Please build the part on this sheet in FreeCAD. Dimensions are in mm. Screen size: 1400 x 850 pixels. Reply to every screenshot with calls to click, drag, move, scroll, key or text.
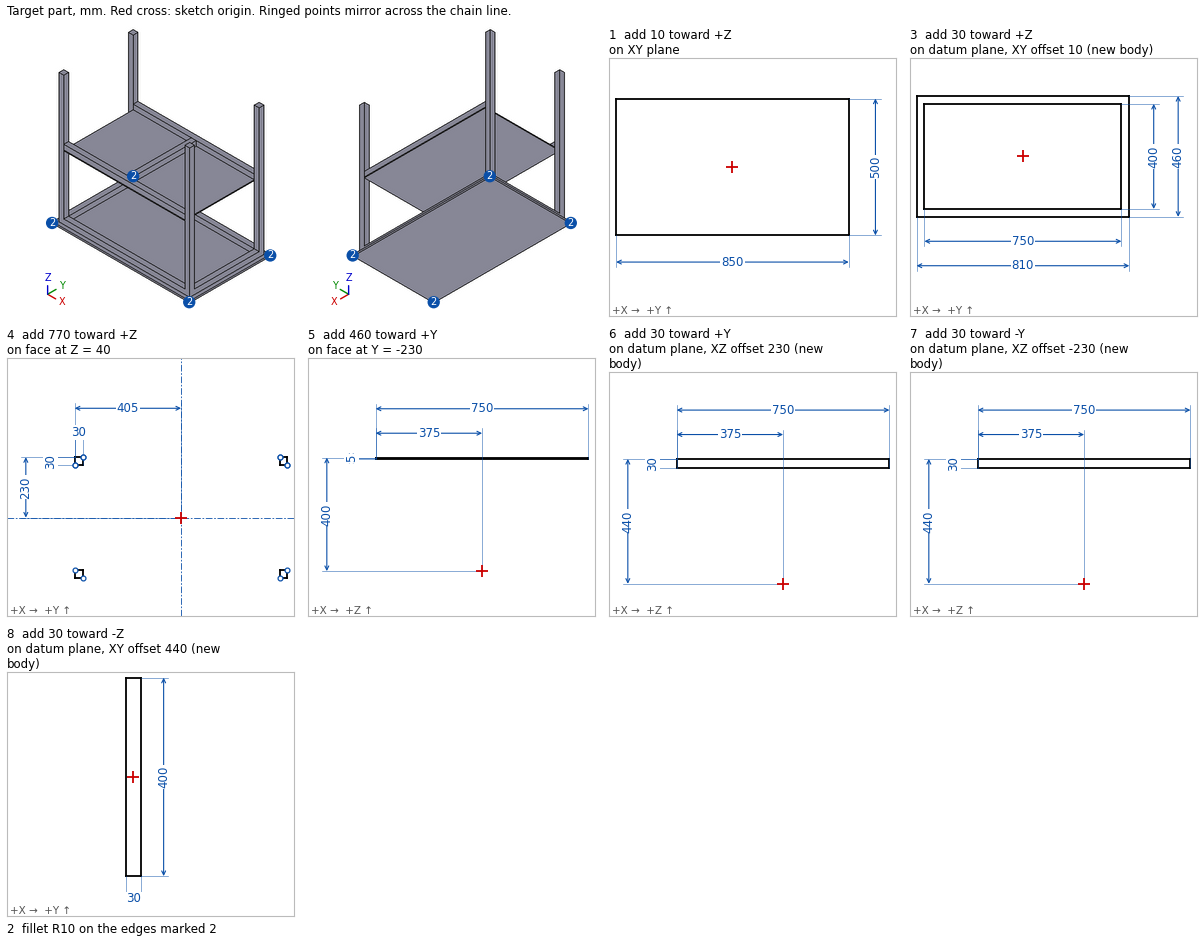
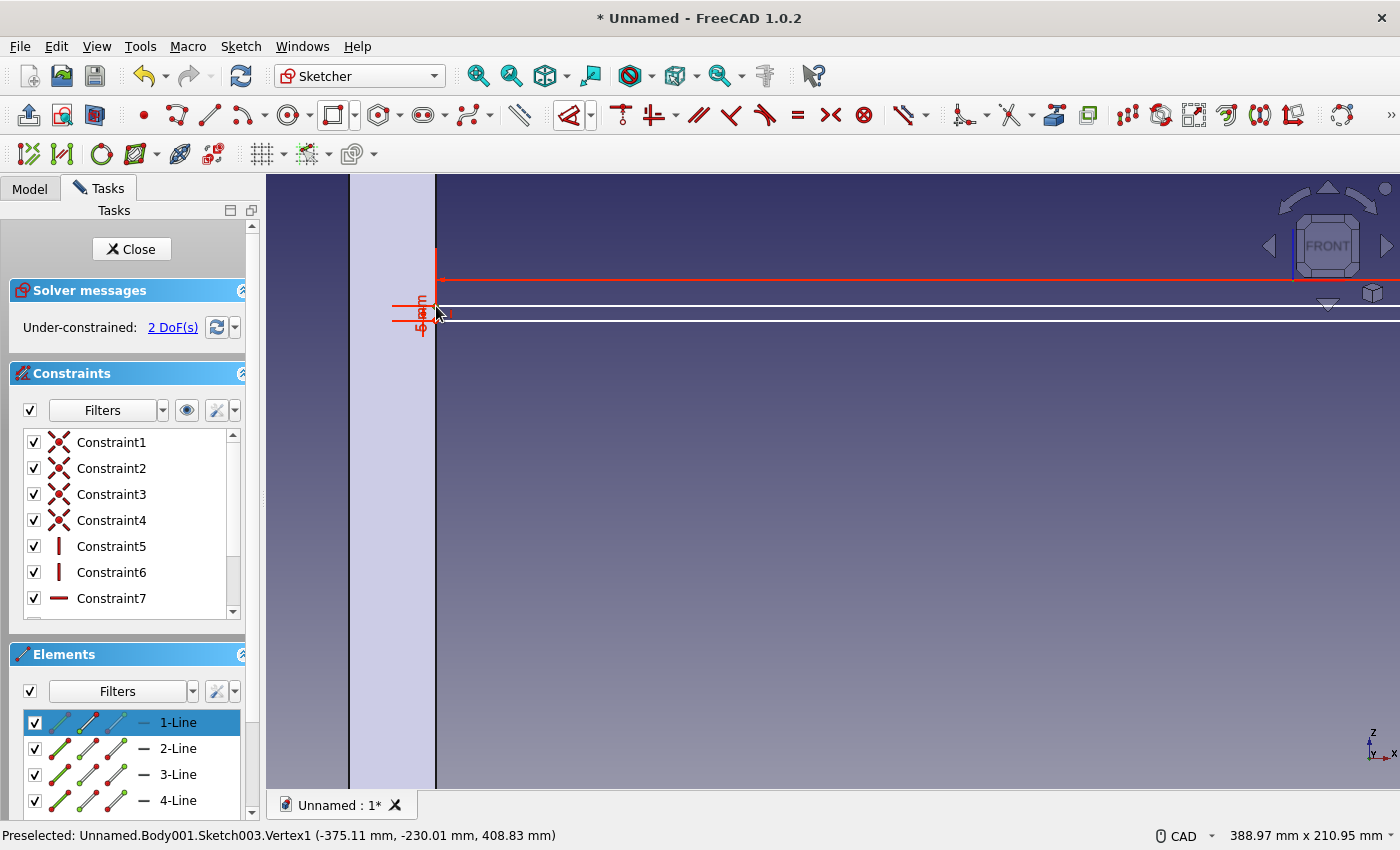
click(590, 116)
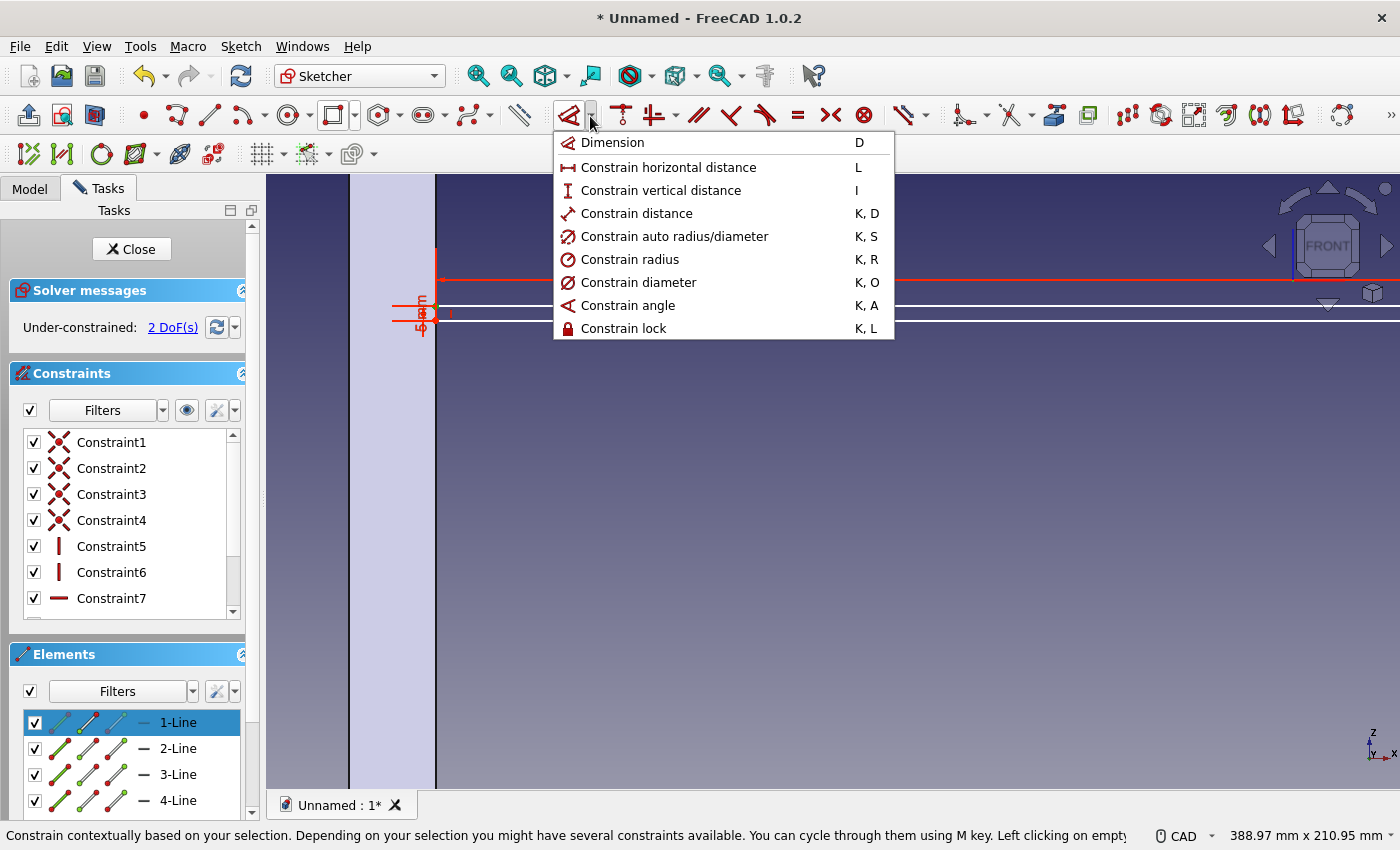
click(724, 168)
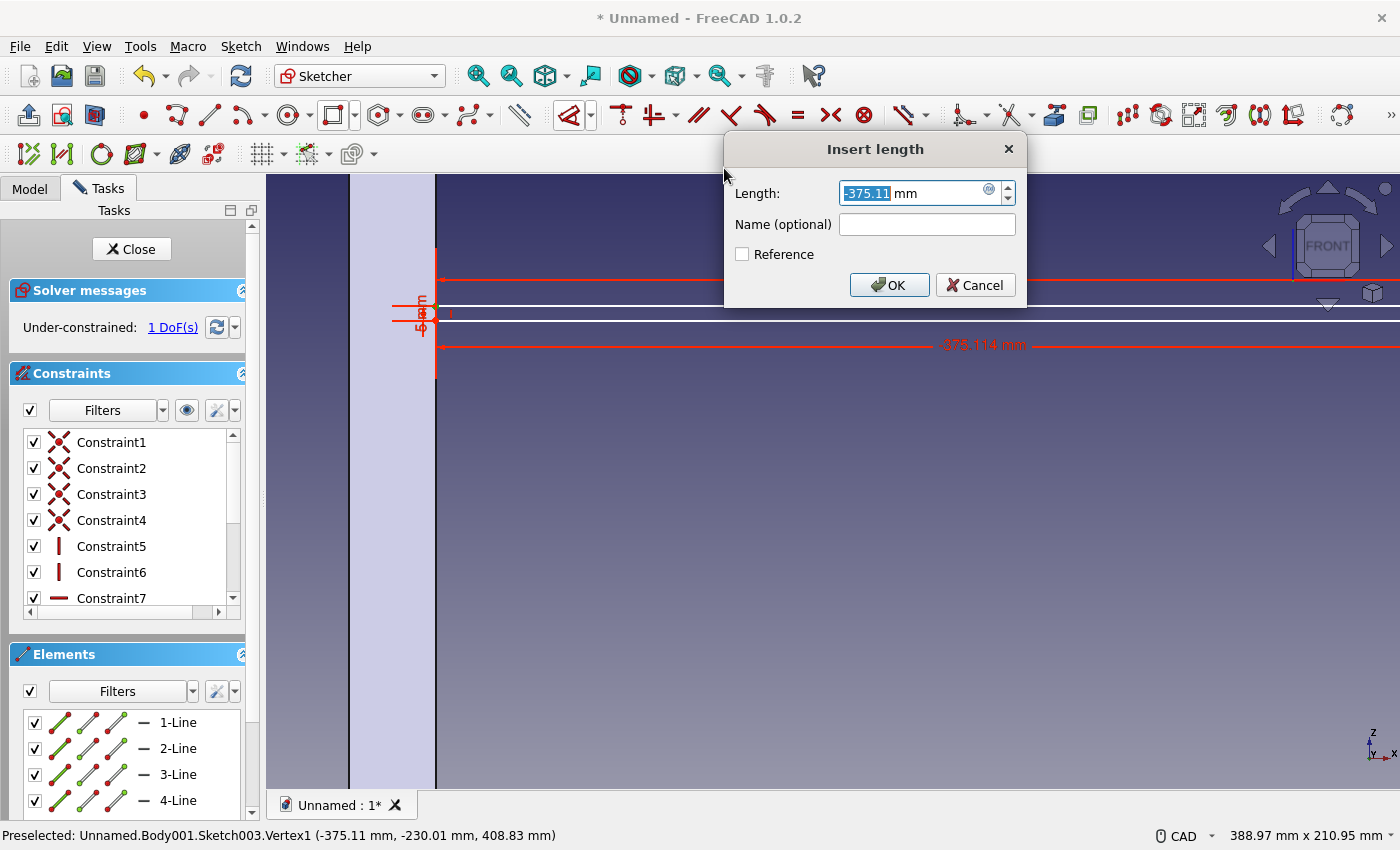
text(-375)
key(Return)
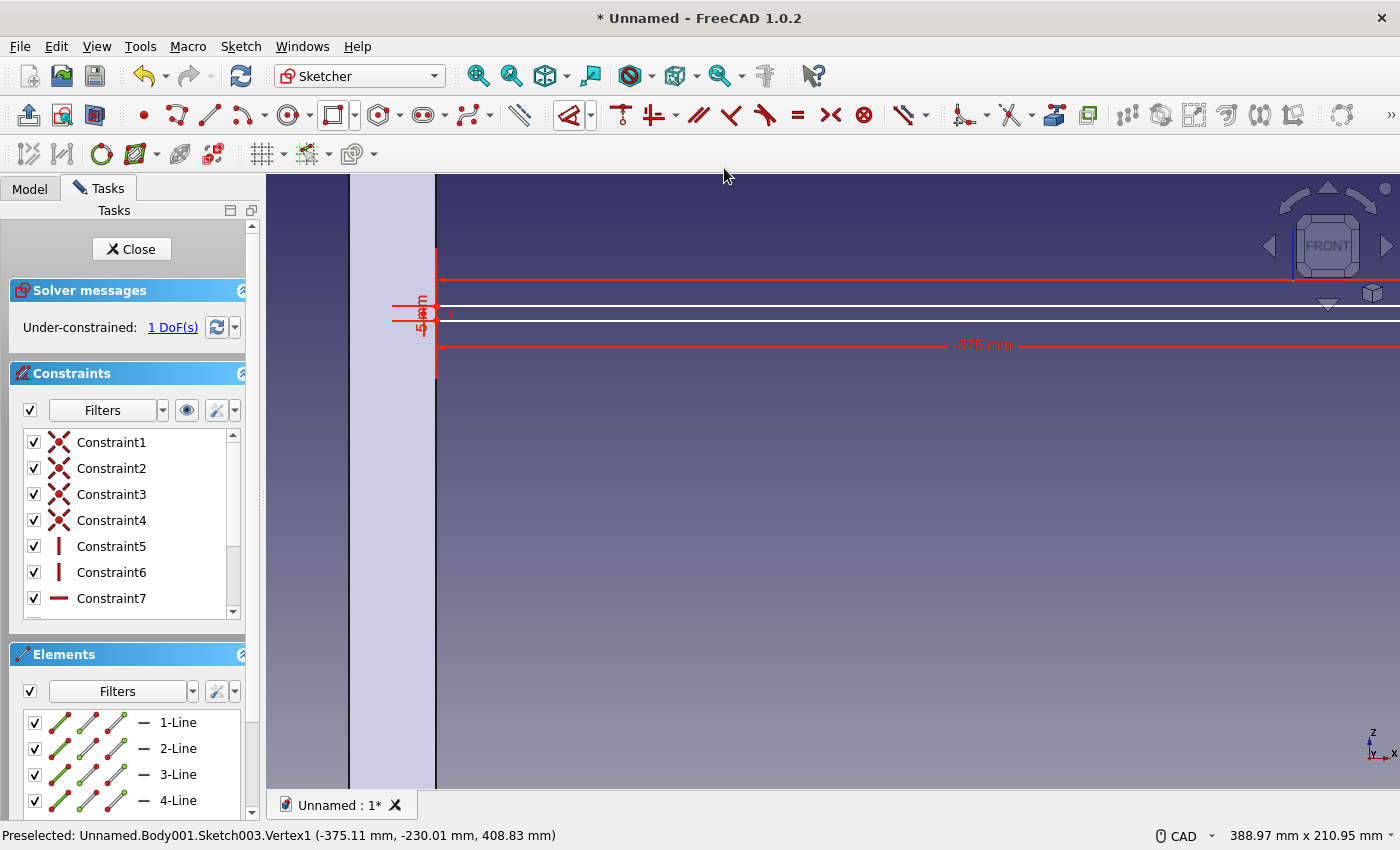
click(436, 306)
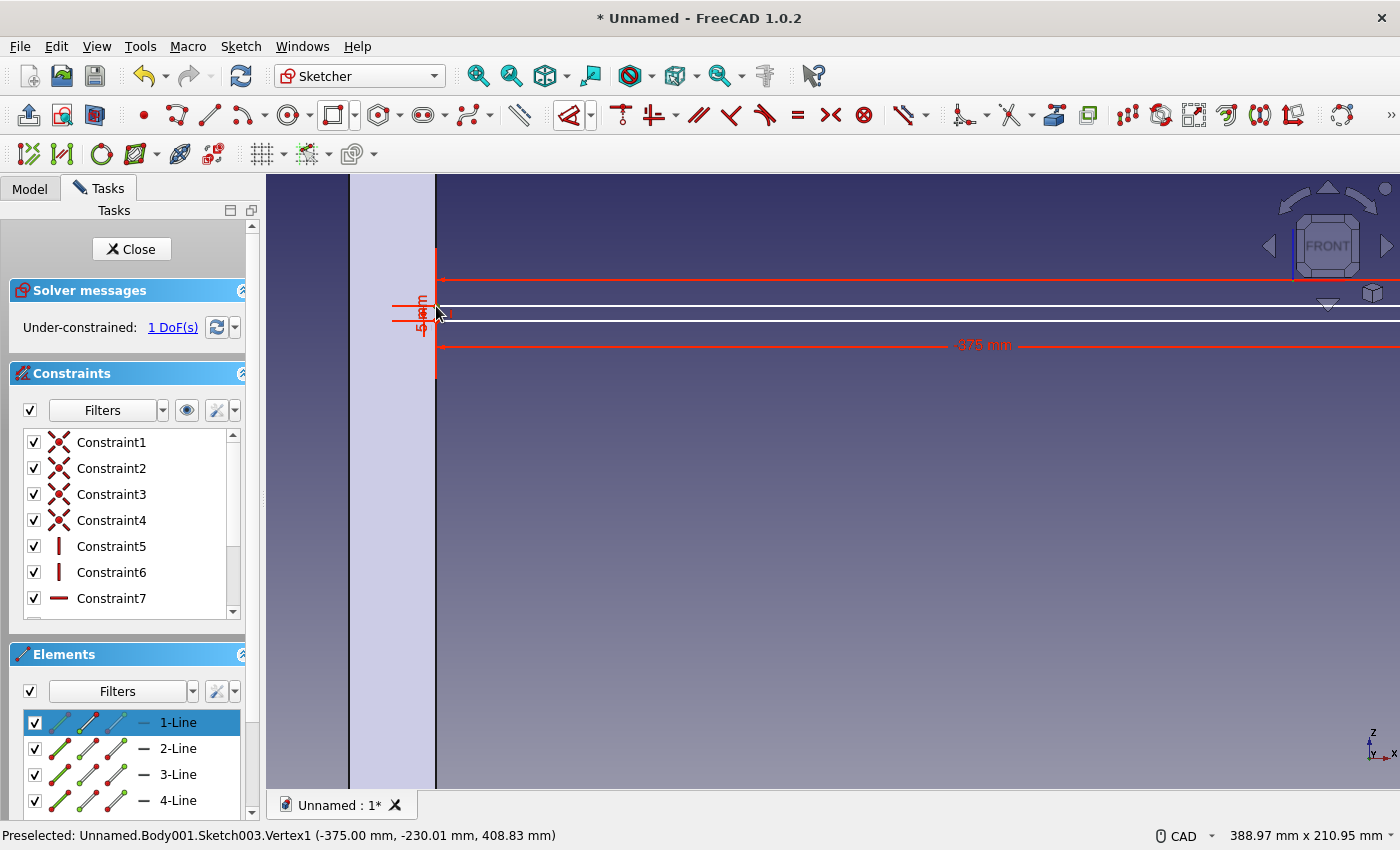
key(i)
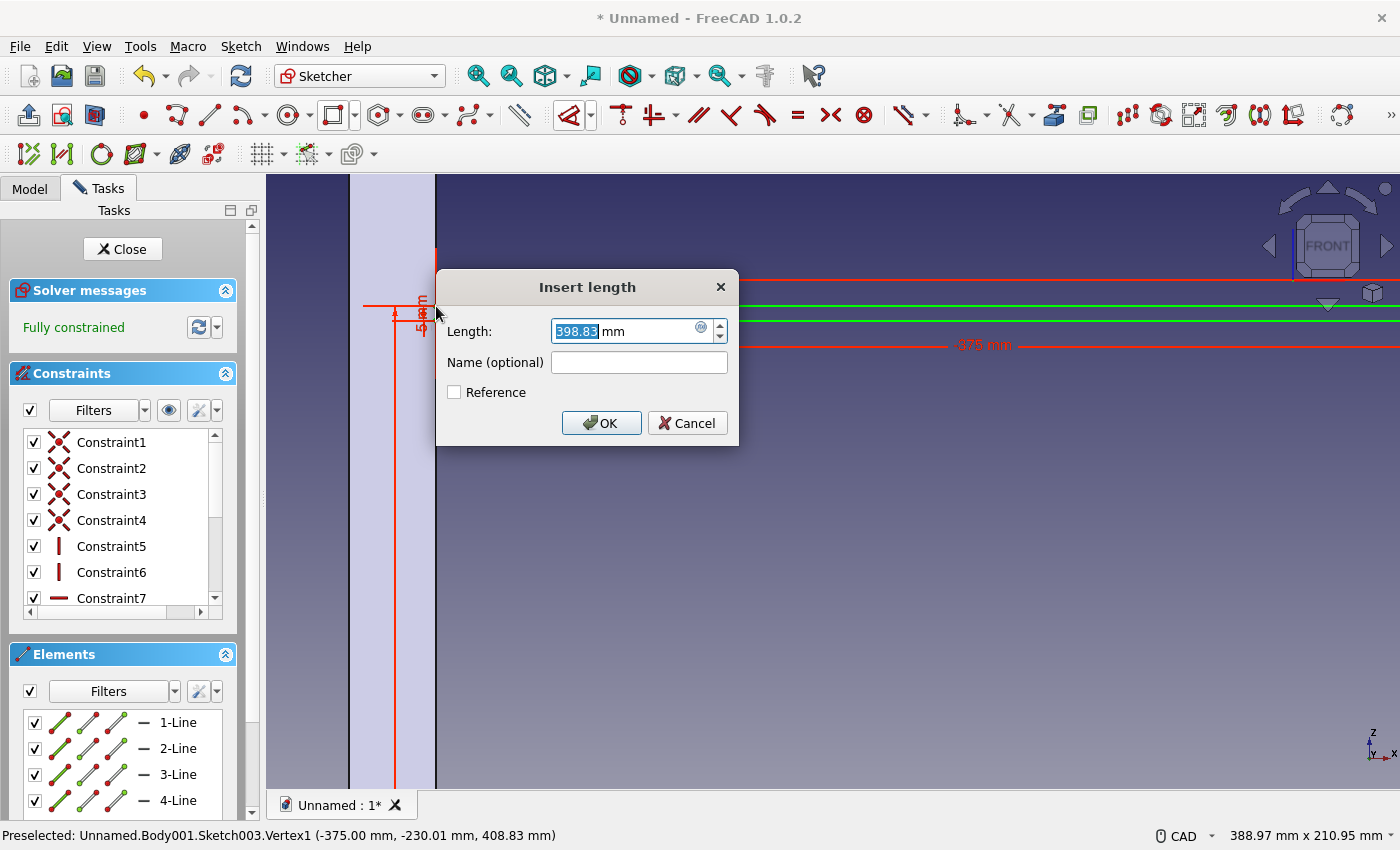
text(400)
key(Return)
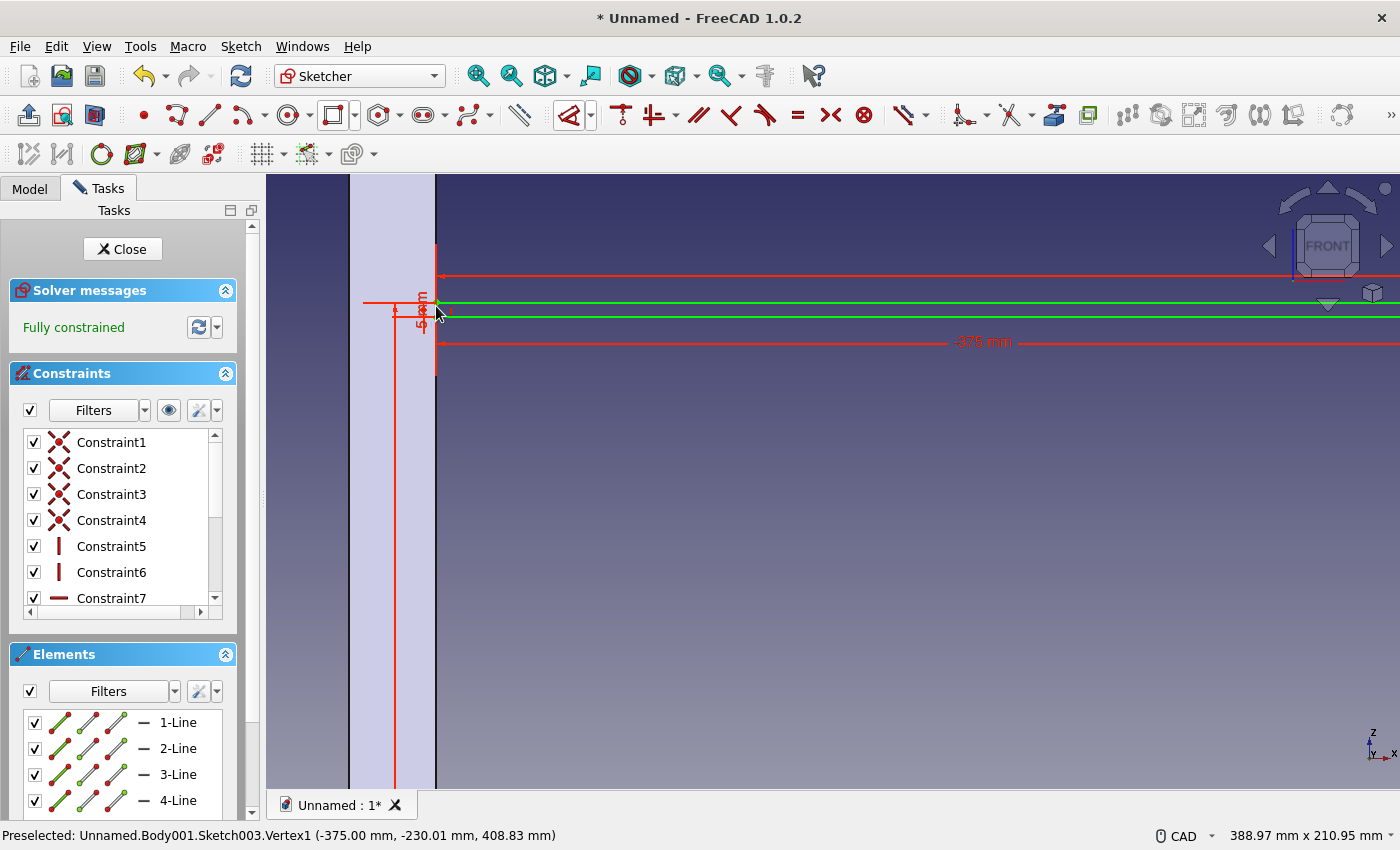
click(123, 249)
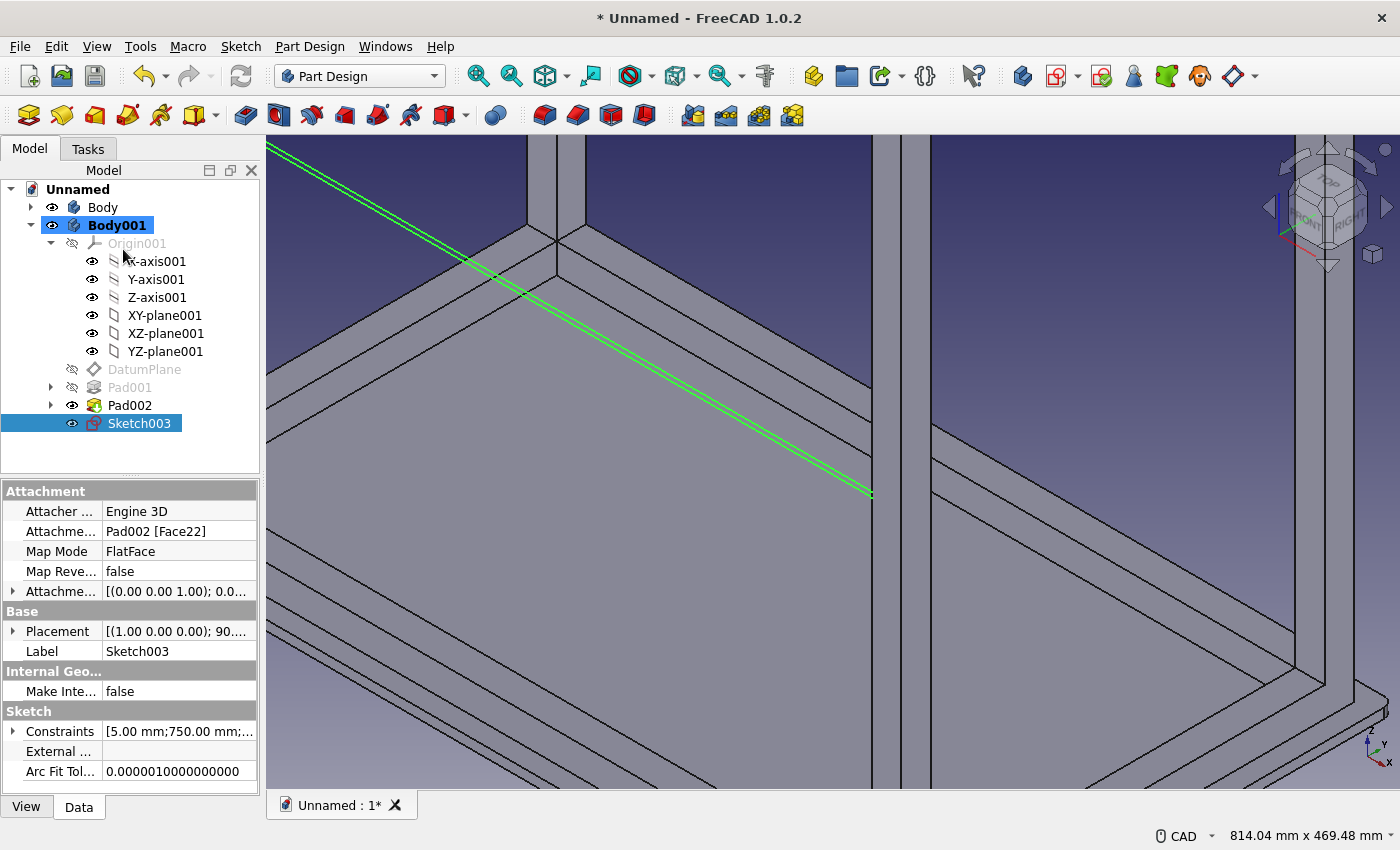
click(29, 116)